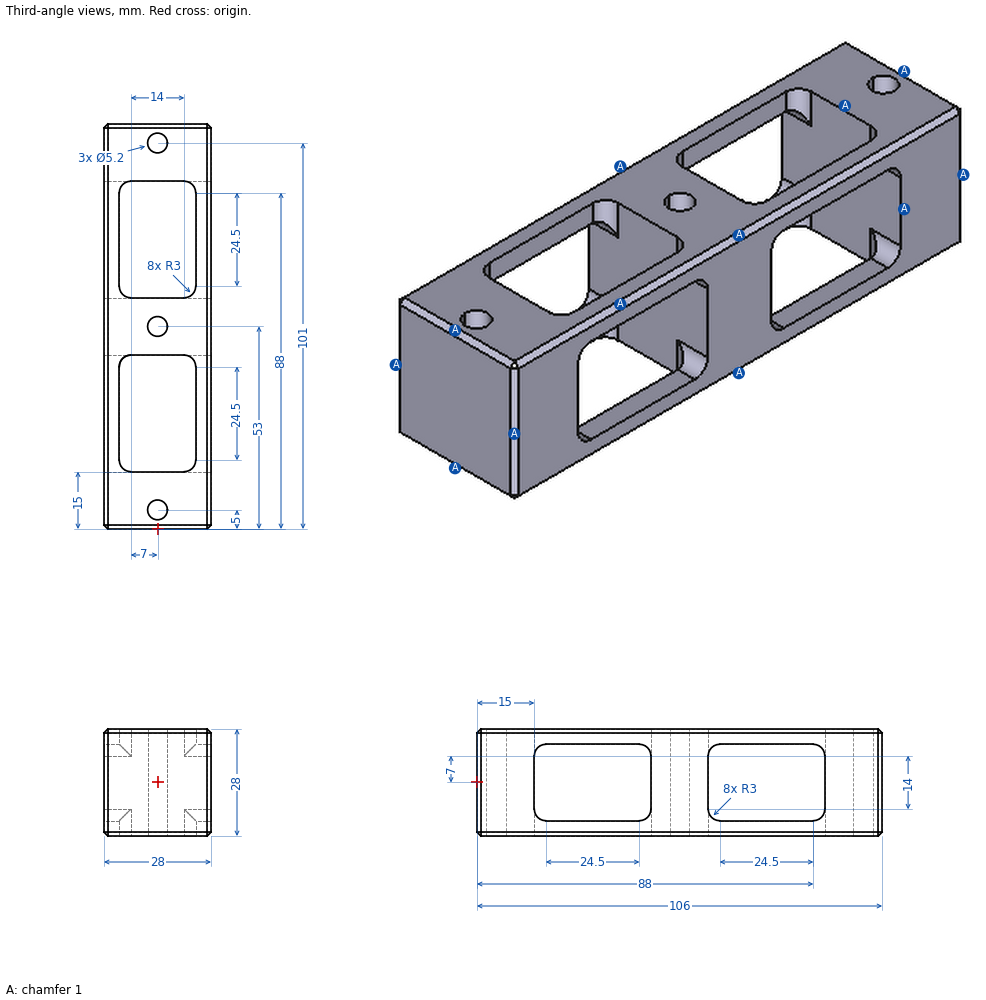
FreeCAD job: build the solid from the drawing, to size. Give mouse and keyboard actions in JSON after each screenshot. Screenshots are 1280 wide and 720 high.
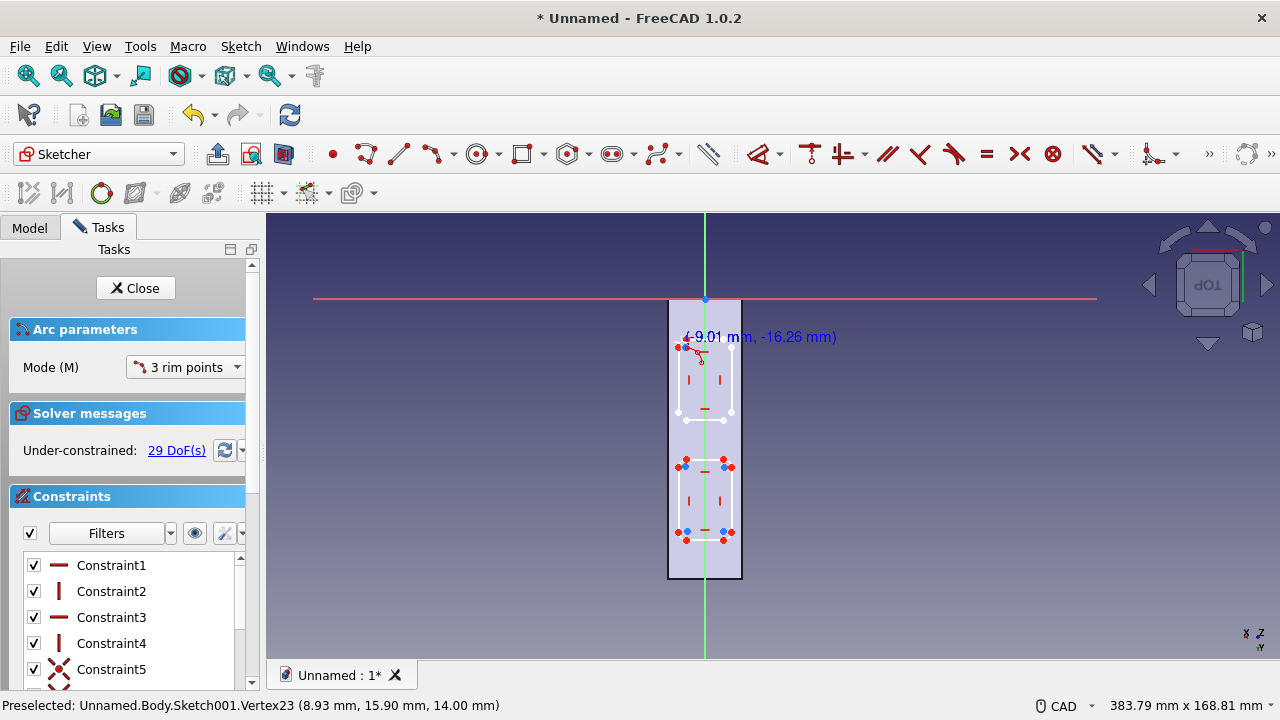
{"action": "scroll", "coordinate": [679, 412], "scroll_direction": "up", "scroll_amount": 2}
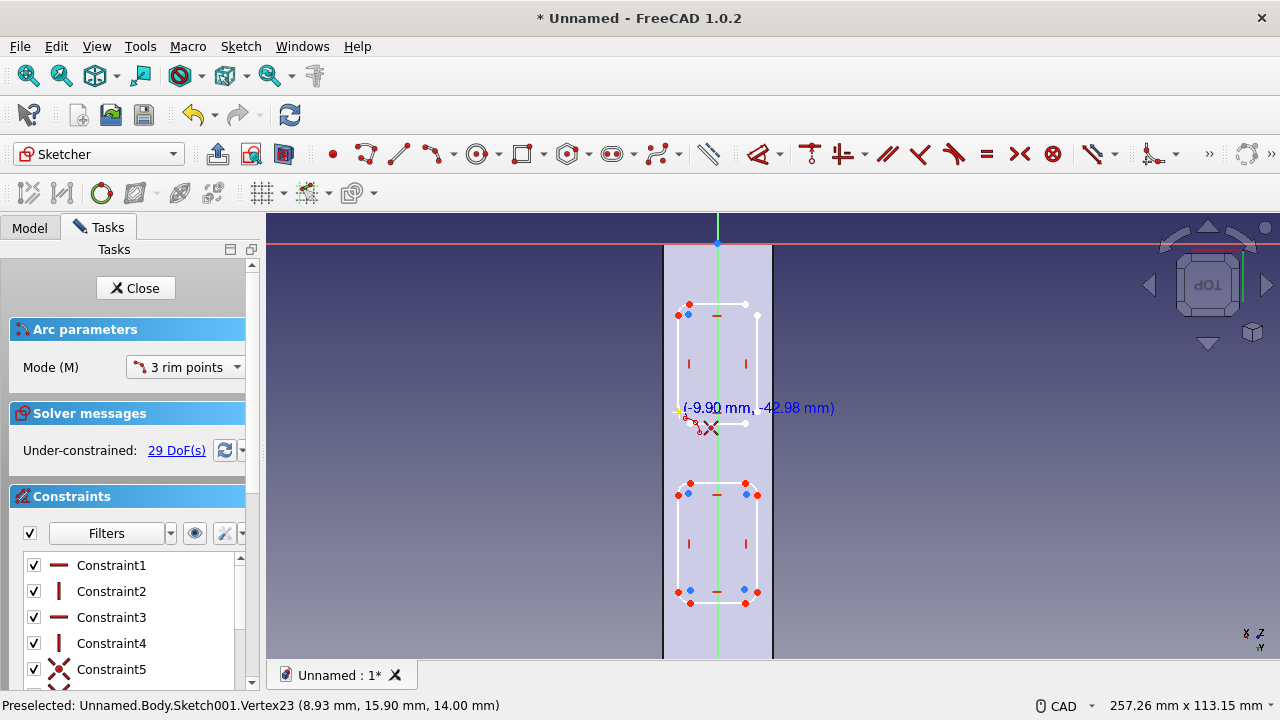
{"action": "left_click", "coordinate": [678, 412]}
{"action": "left_click", "coordinate": [690, 424]}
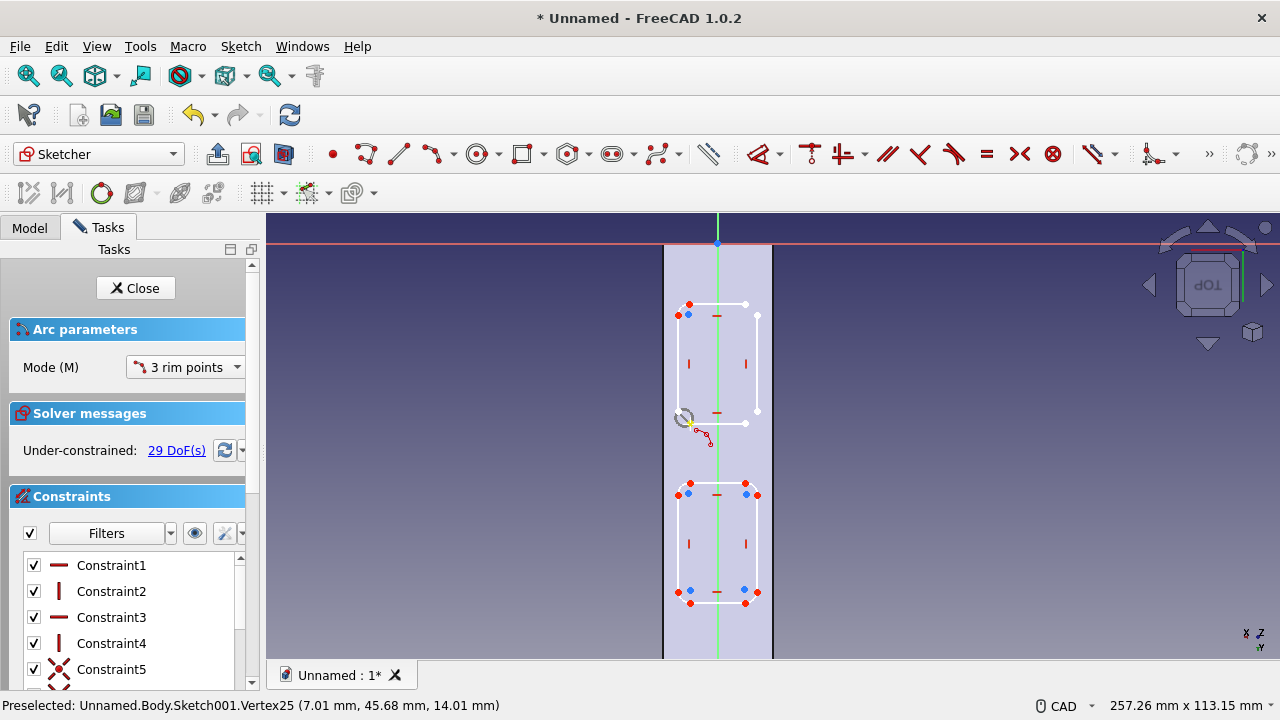
{"action": "scroll", "coordinate": [682, 420], "scroll_direction": "up", "scroll_amount": 8}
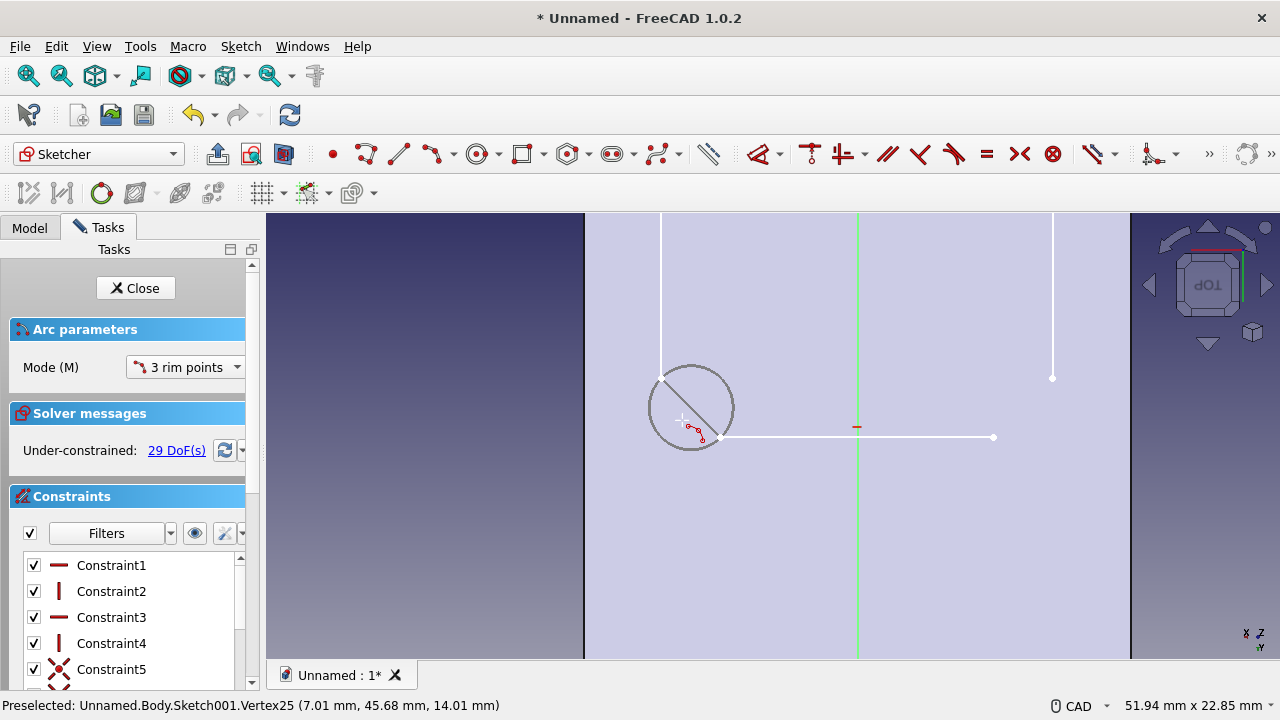
{"action": "left_click", "coordinate": [680, 417]}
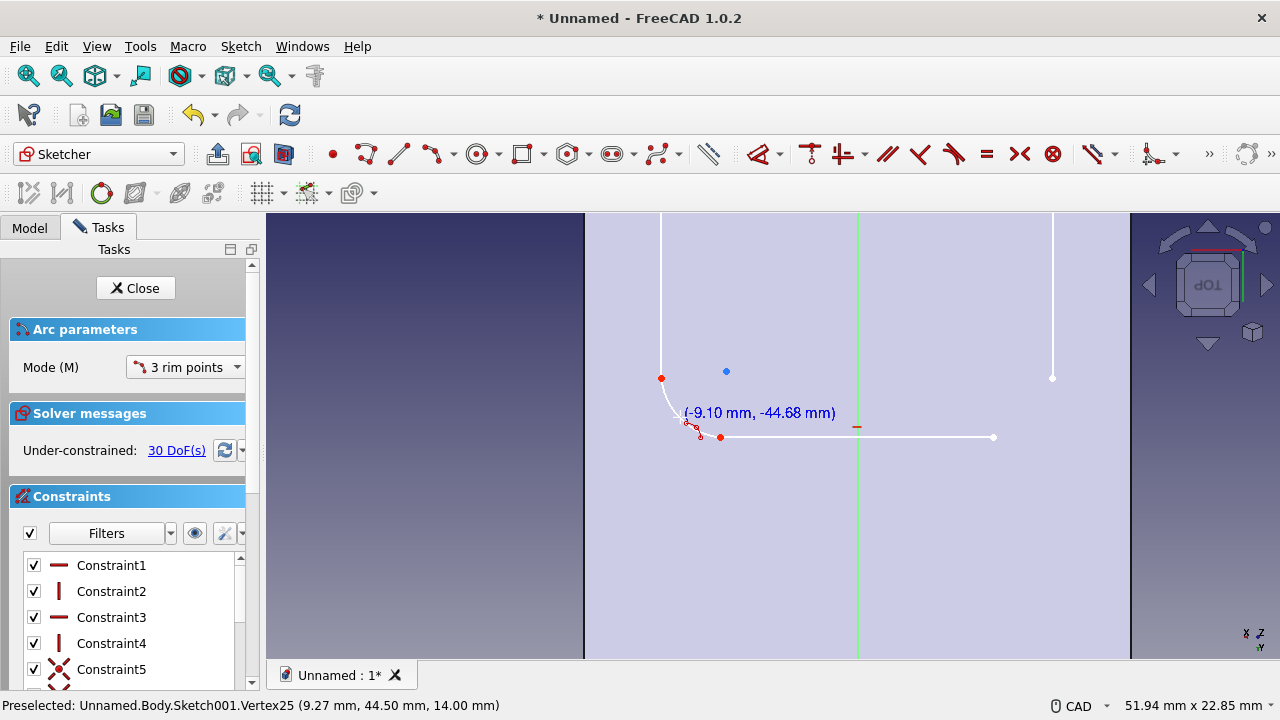
{"action": "scroll", "coordinate": [681, 417], "scroll_direction": "down", "scroll_amount": 10}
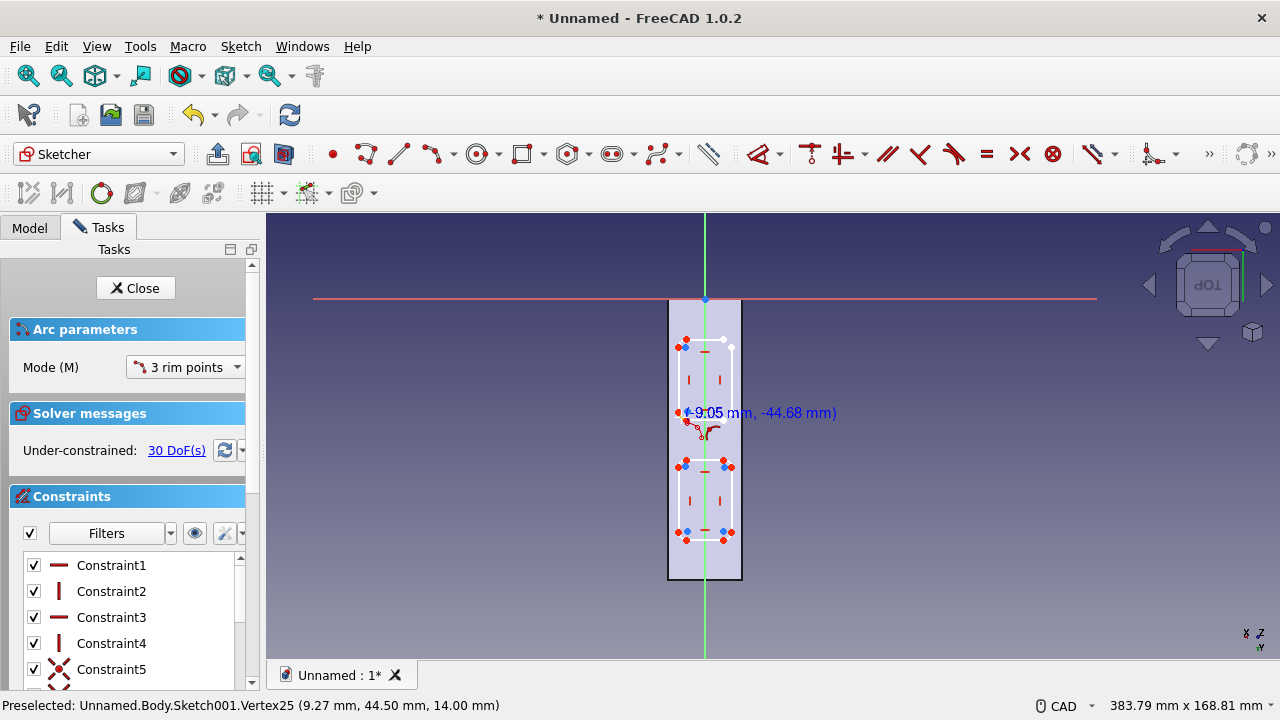
{"action": "scroll", "coordinate": [724, 420], "scroll_direction": "up", "scroll_amount": 2}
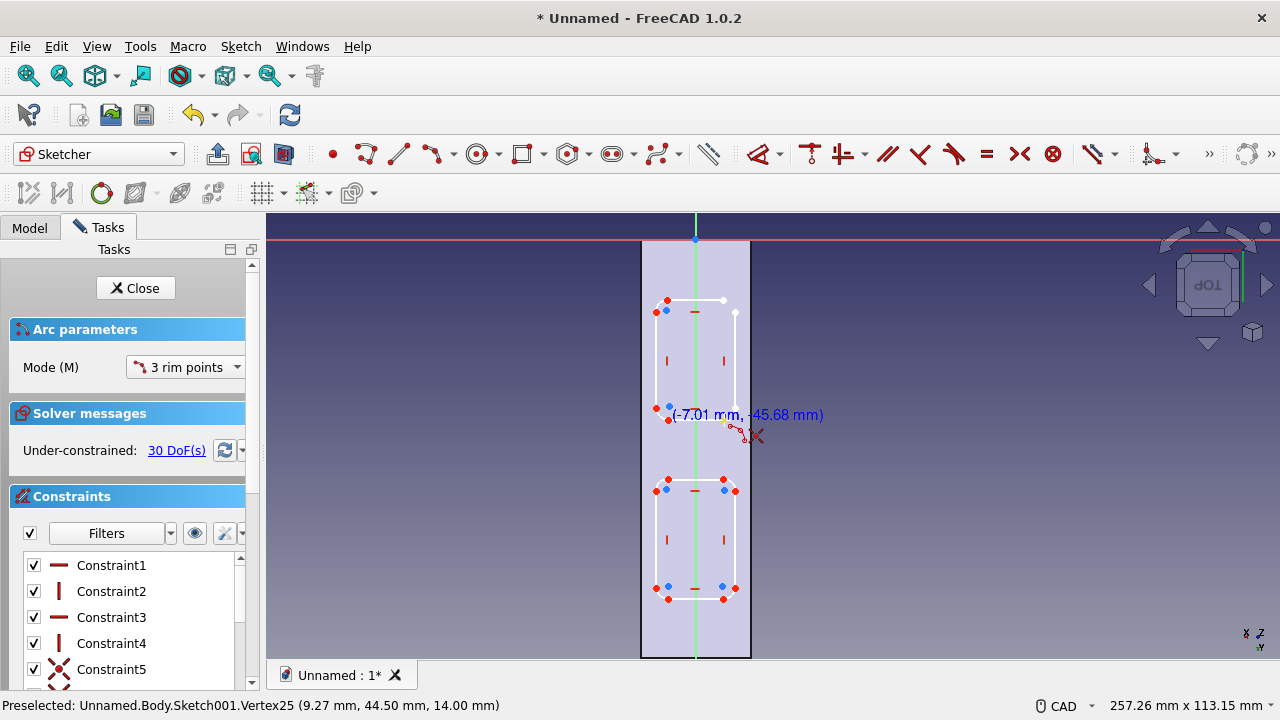
{"action": "left_click", "coordinate": [723, 420]}
{"action": "left_click", "coordinate": [735, 408]}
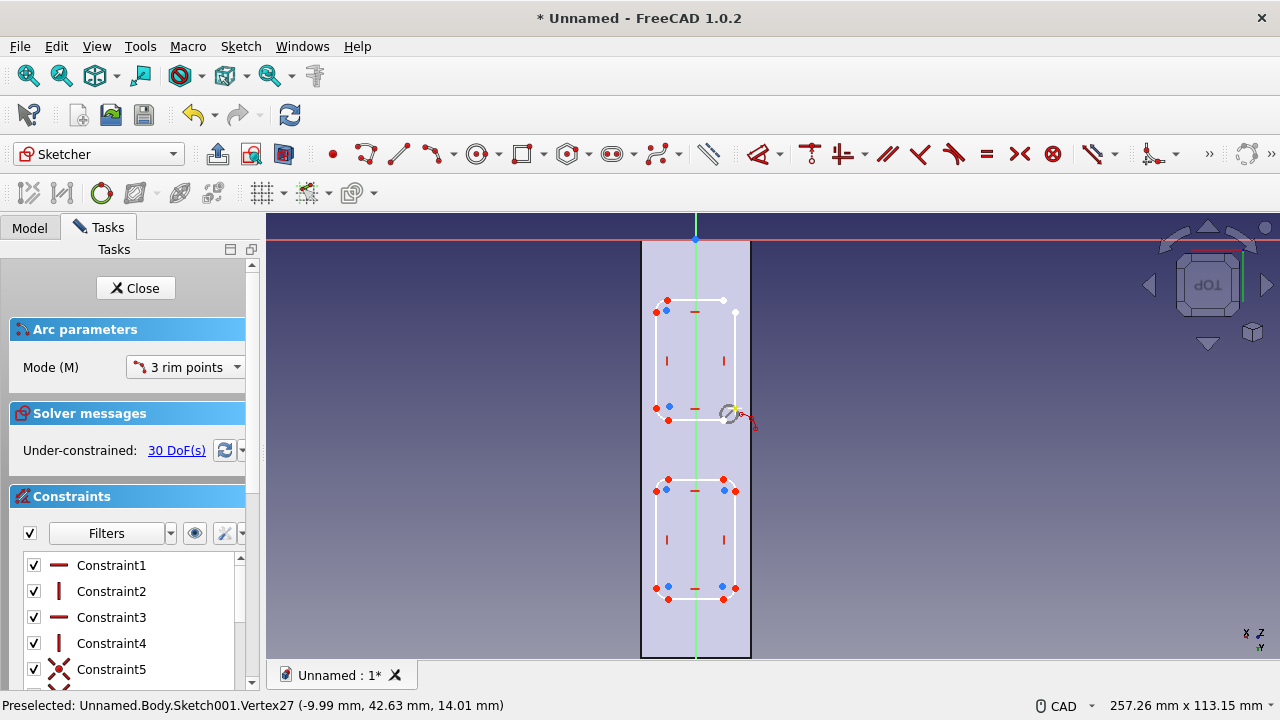
{"action": "scroll", "coordinate": [732, 416], "scroll_direction": "up", "scroll_amount": 8}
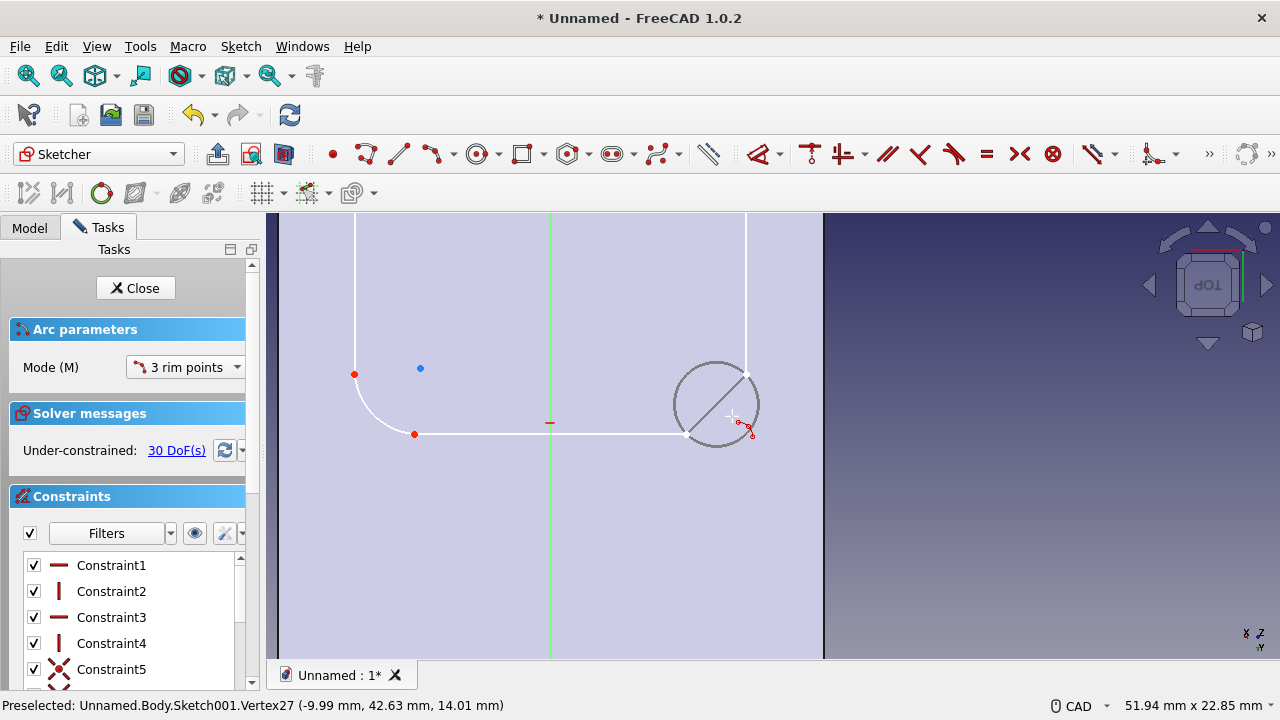
{"action": "left_click", "coordinate": [729, 413]}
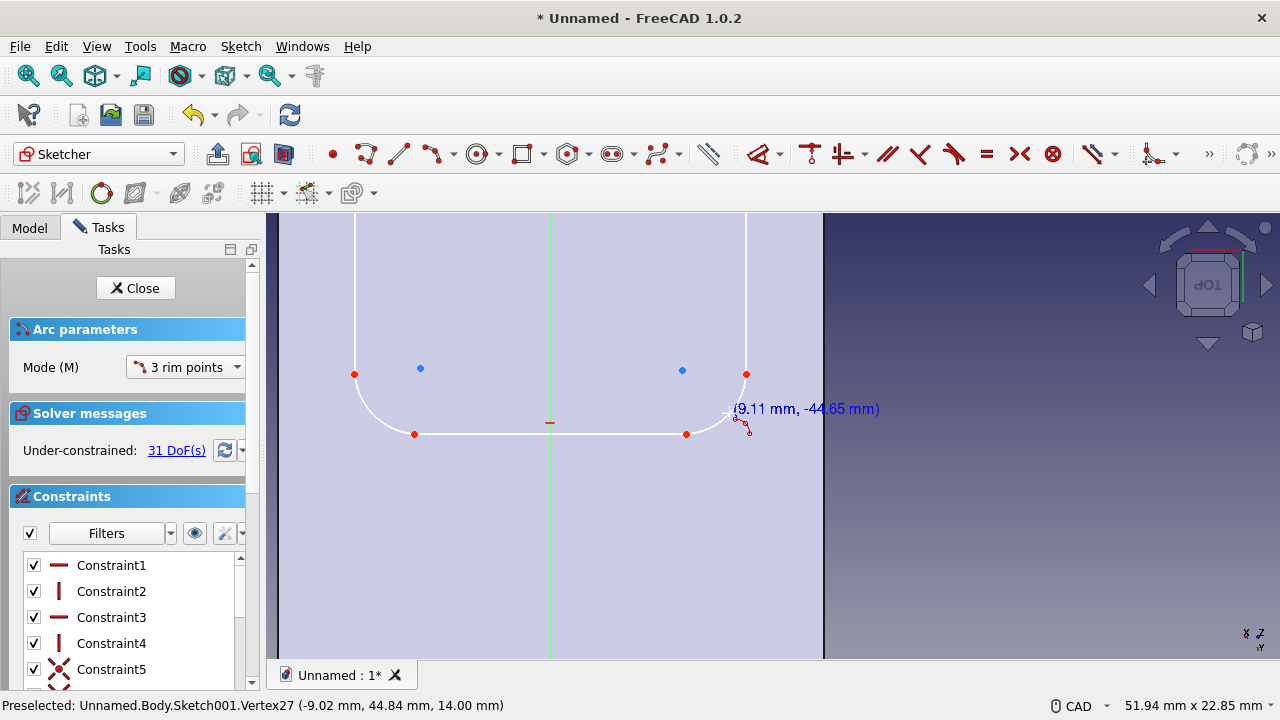
{"action": "scroll", "coordinate": [729, 418], "scroll_direction": "down", "scroll_amount": 10}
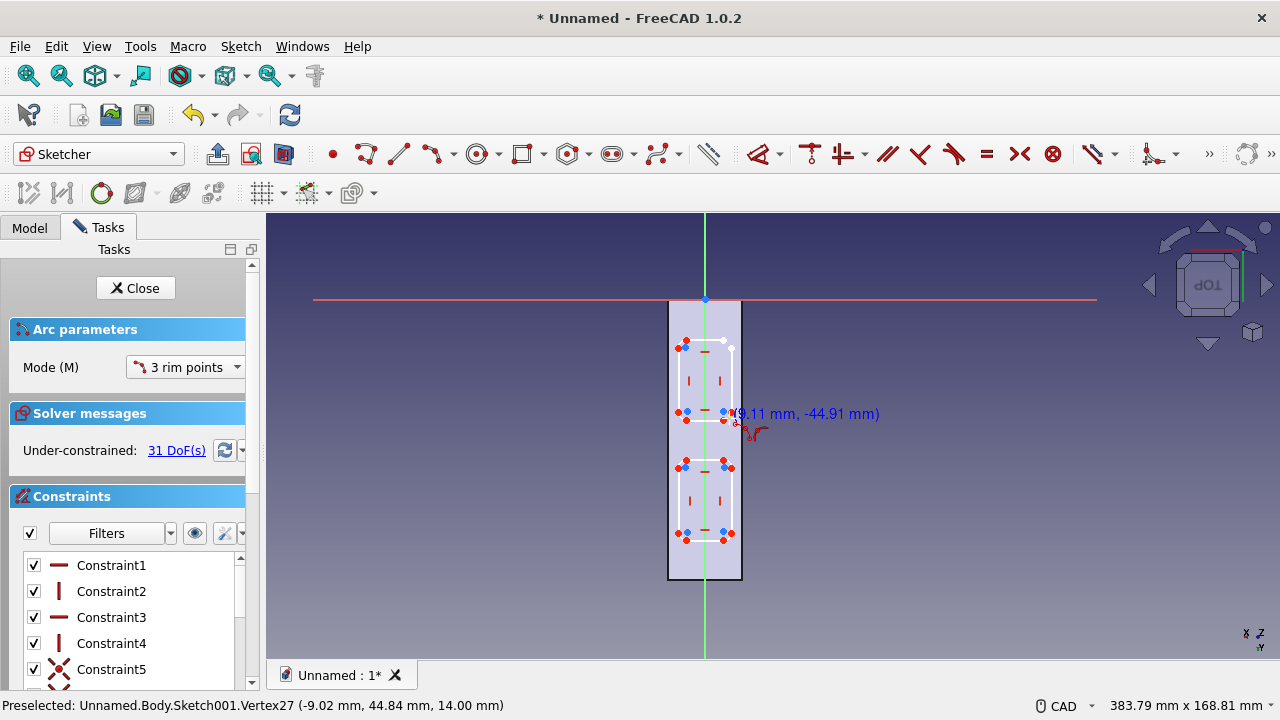
{"action": "scroll", "coordinate": [732, 347], "scroll_direction": "up", "scroll_amount": 2}